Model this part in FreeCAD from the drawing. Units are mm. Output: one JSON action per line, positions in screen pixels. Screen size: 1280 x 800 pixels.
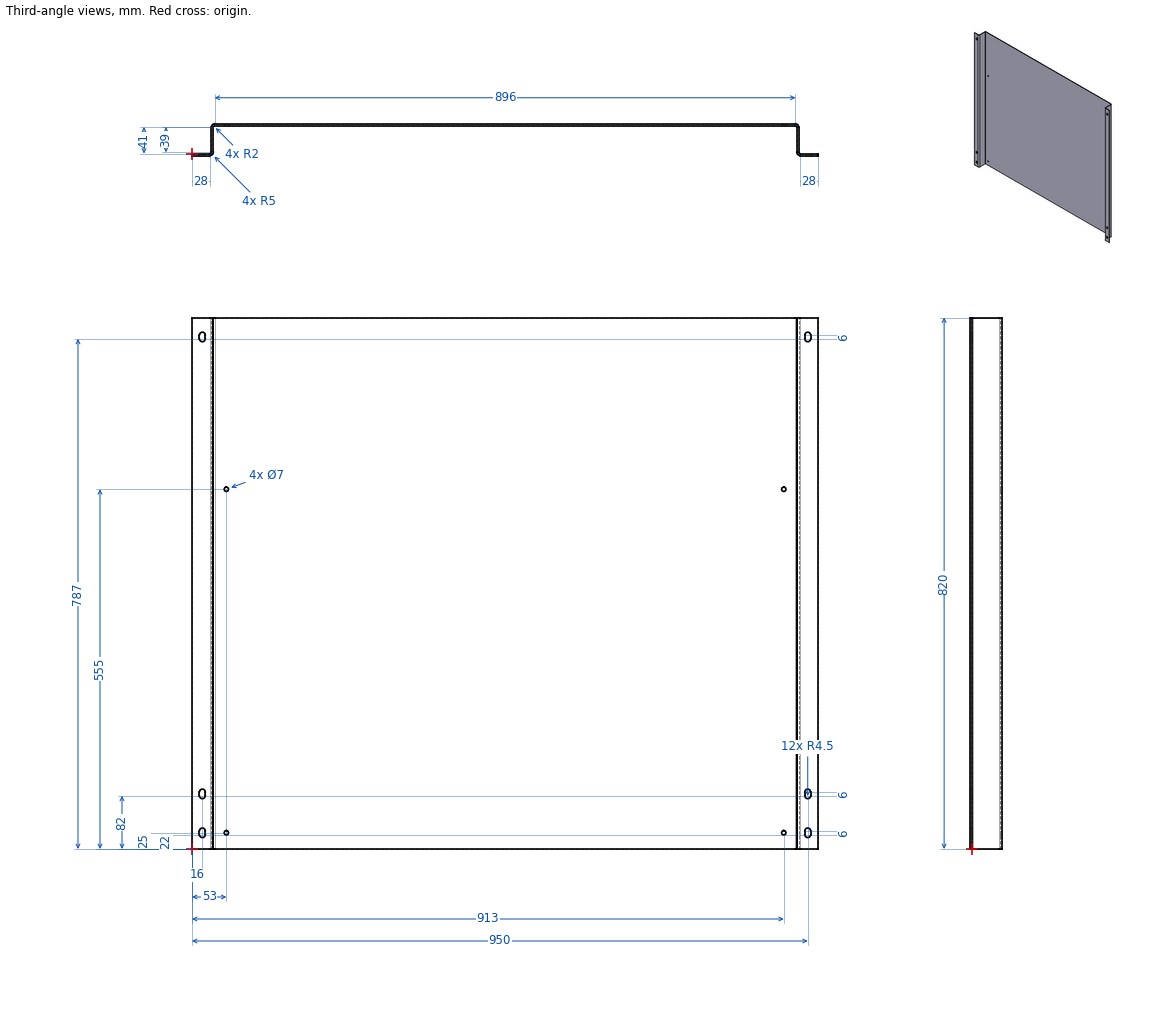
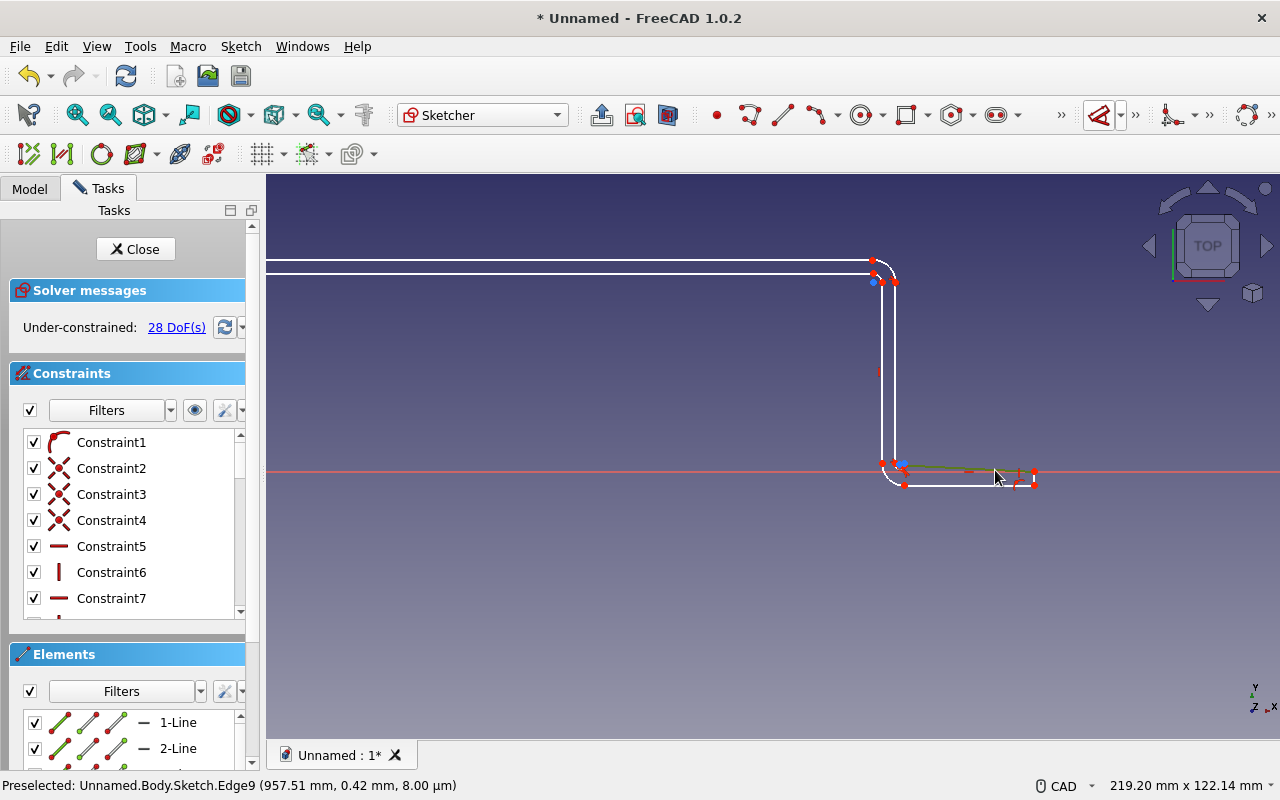
{"action": "scroll", "coordinate": [899, 469], "scroll_direction": "up", "scroll_amount": 4}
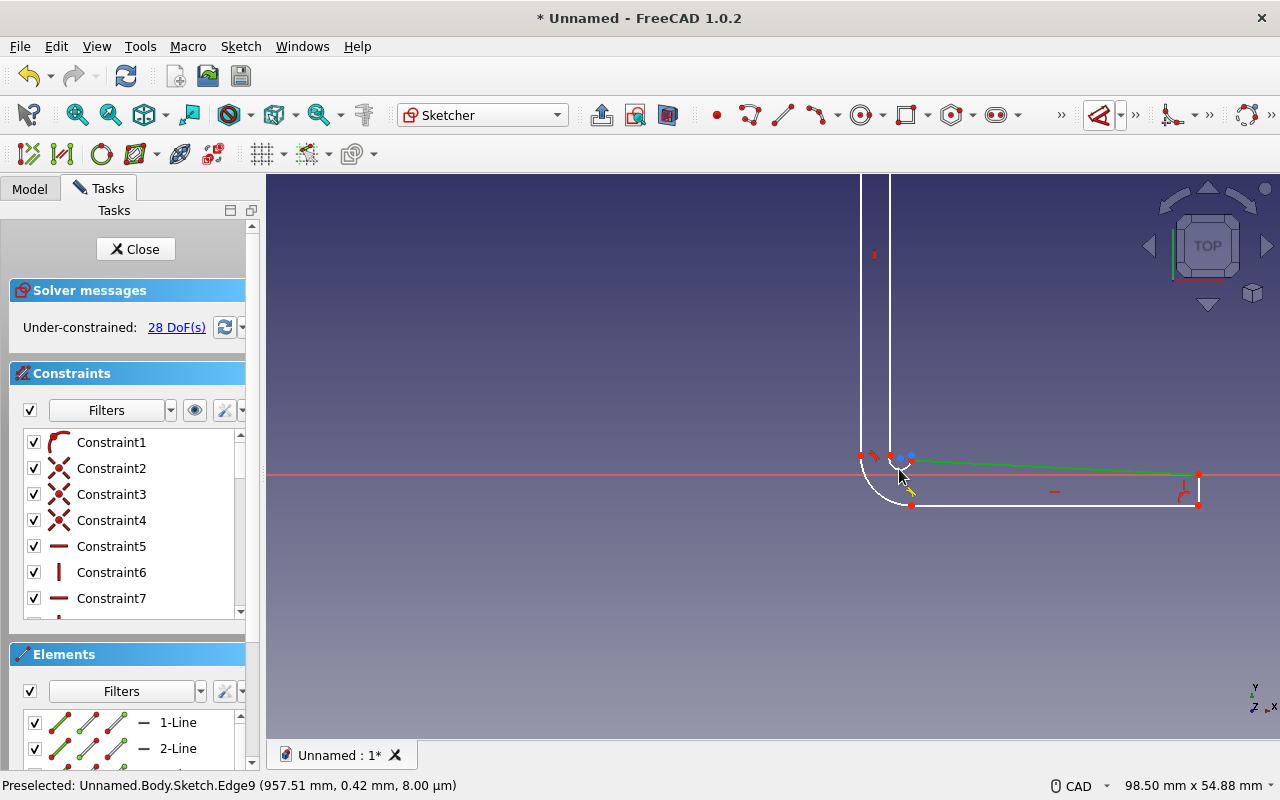
{"action": "left_click", "coordinate": [898, 469]}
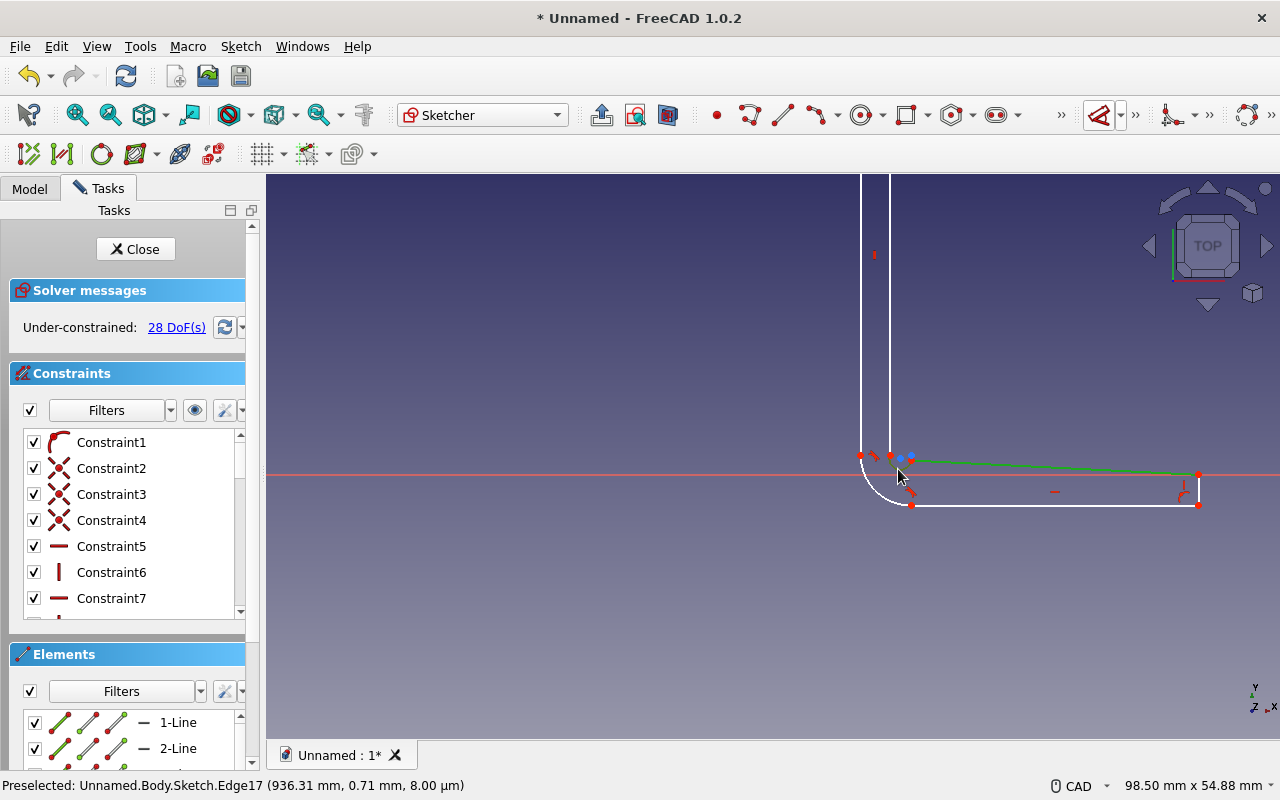
{"action": "key", "text": "t"}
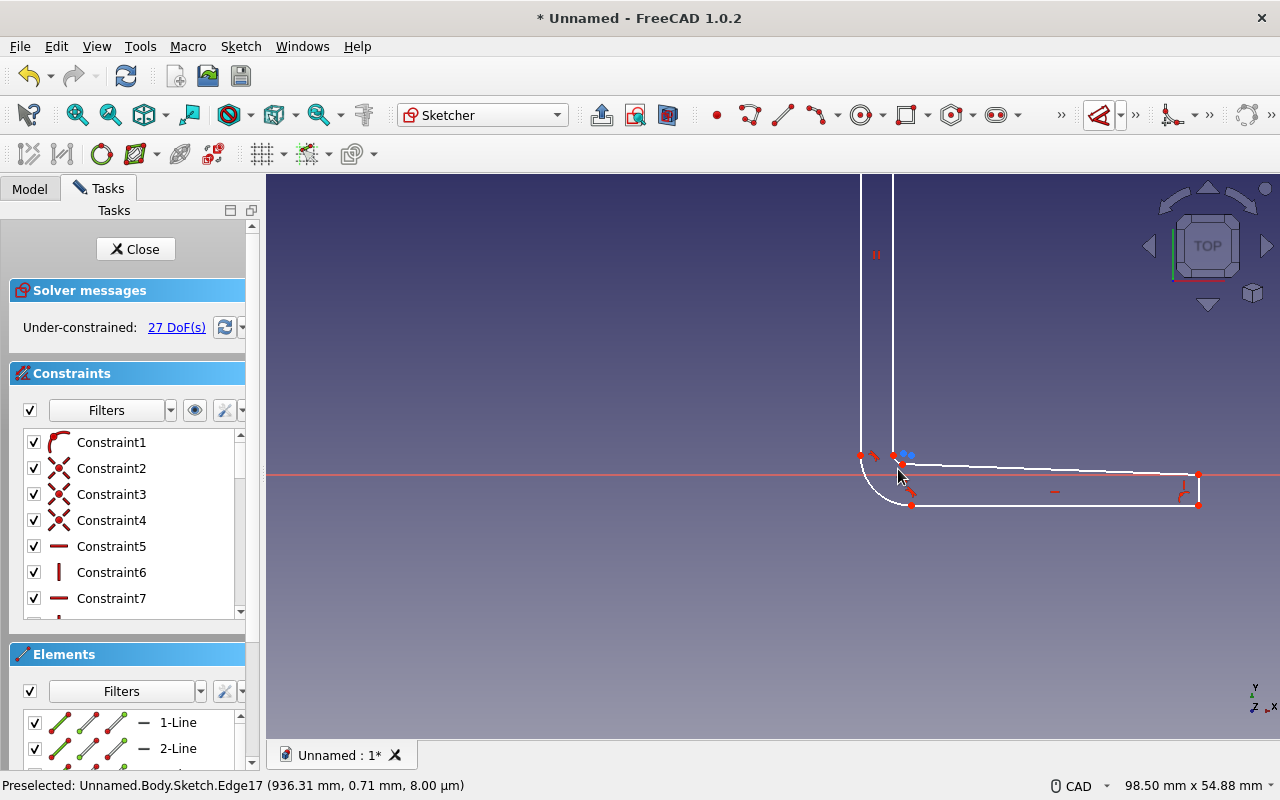
{"action": "left_click", "coordinate": [893, 335]}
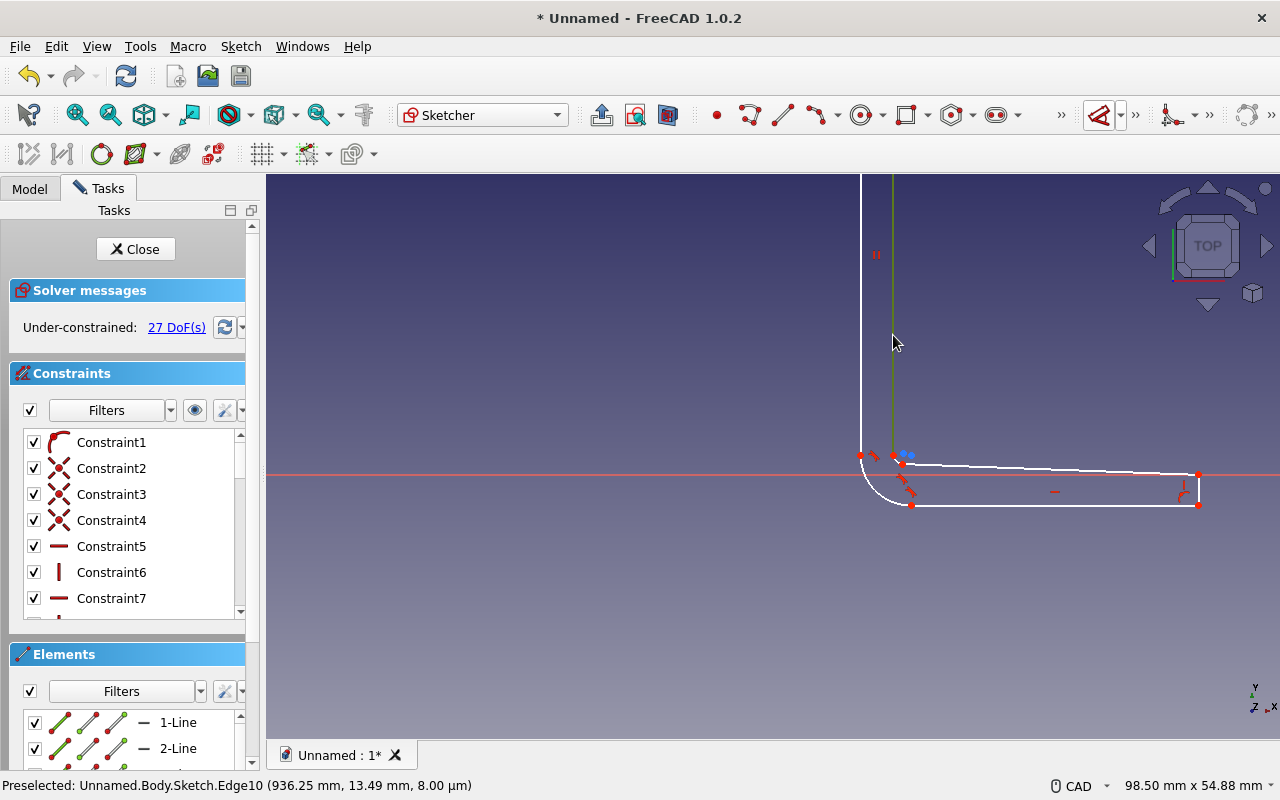
{"action": "left_click", "coordinate": [896, 461]}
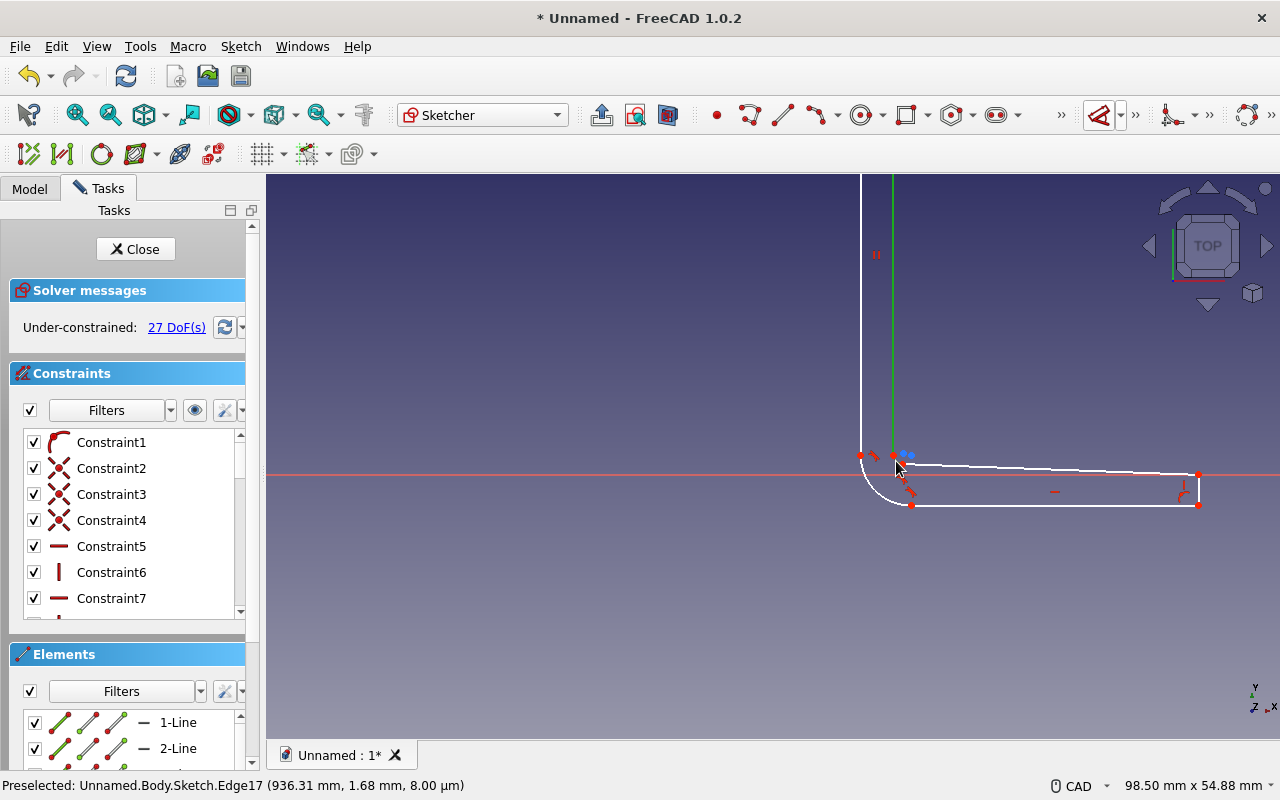
{"action": "key", "text": "t"}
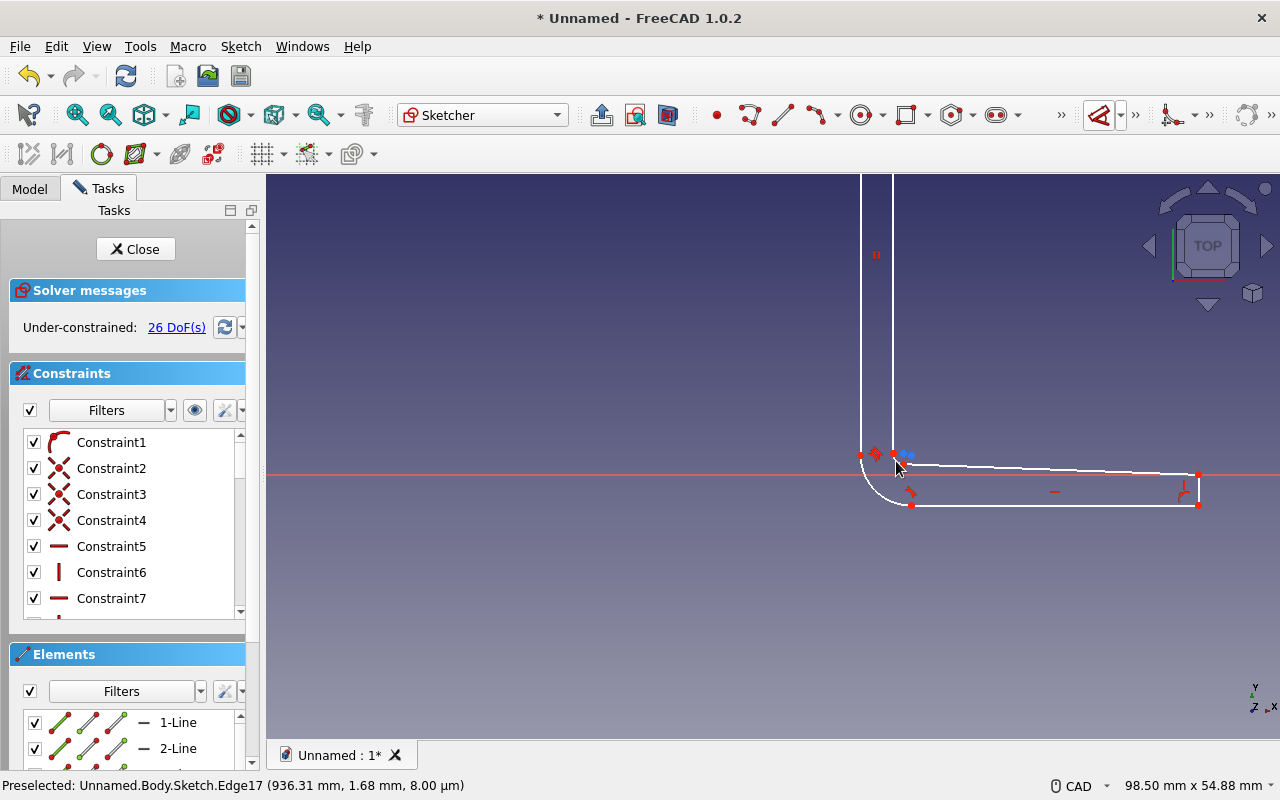
{"action": "left_click", "coordinate": [893, 334]}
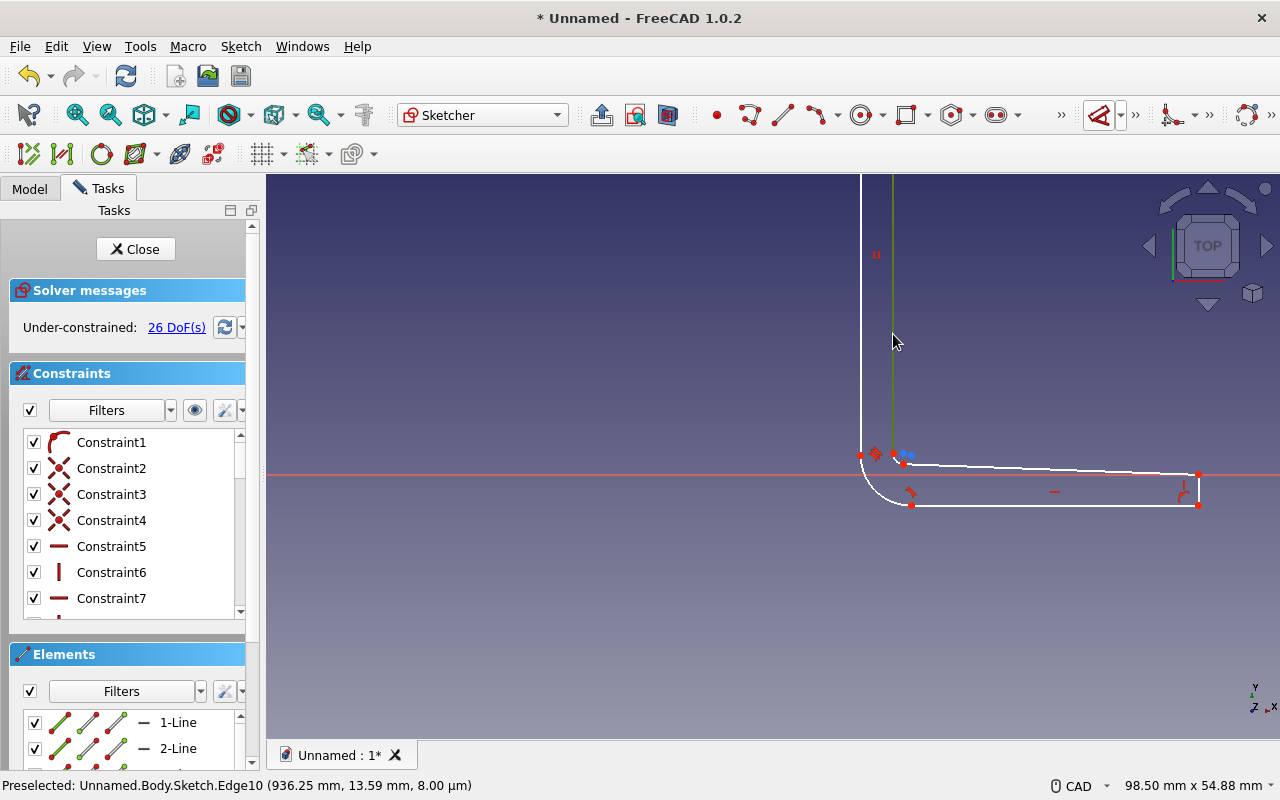
{"action": "scroll", "coordinate": [994, 470], "scroll_direction": "down", "scroll_amount": 14}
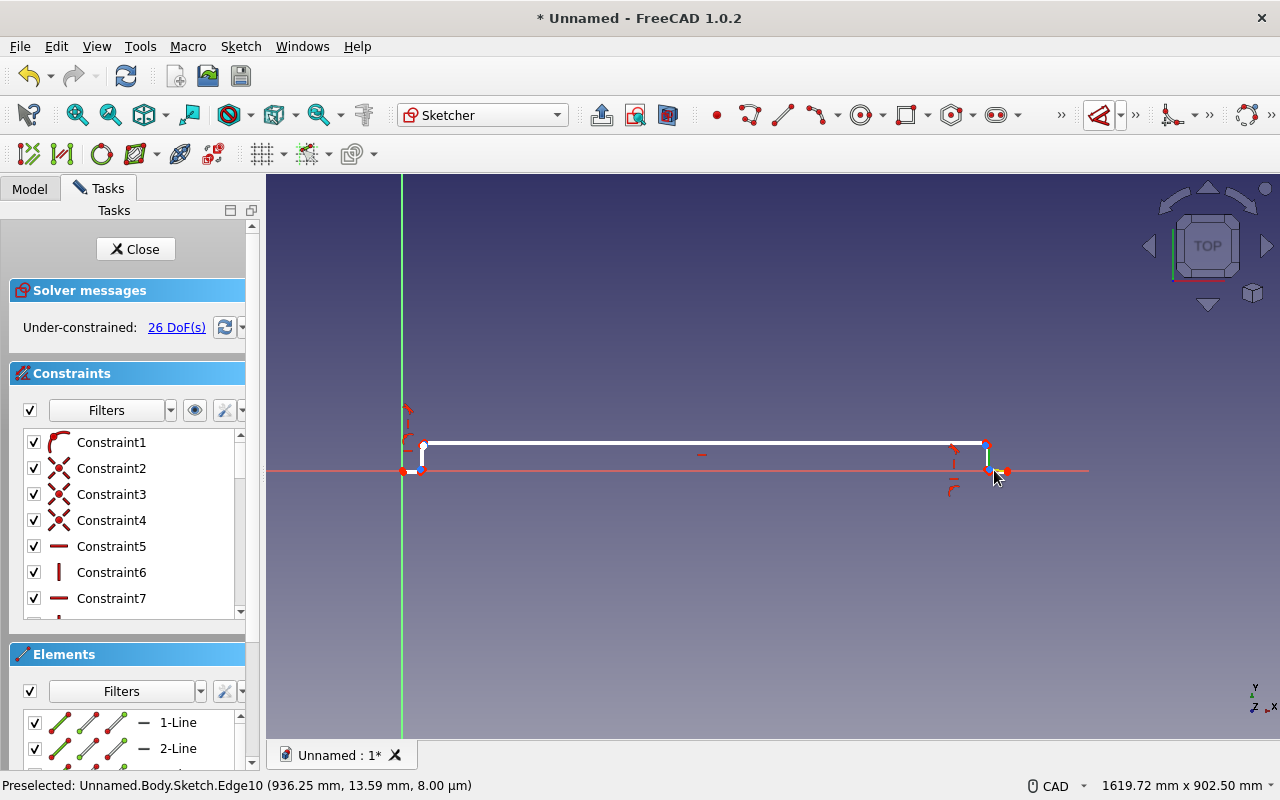
{"action": "scroll", "coordinate": [988, 444], "scroll_direction": "up", "scroll_amount": 12}